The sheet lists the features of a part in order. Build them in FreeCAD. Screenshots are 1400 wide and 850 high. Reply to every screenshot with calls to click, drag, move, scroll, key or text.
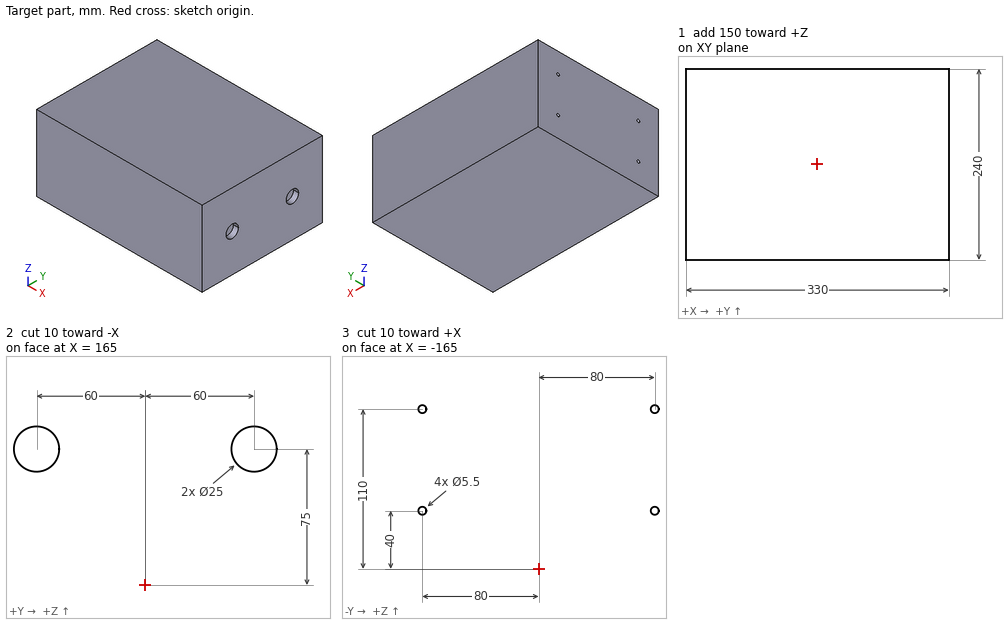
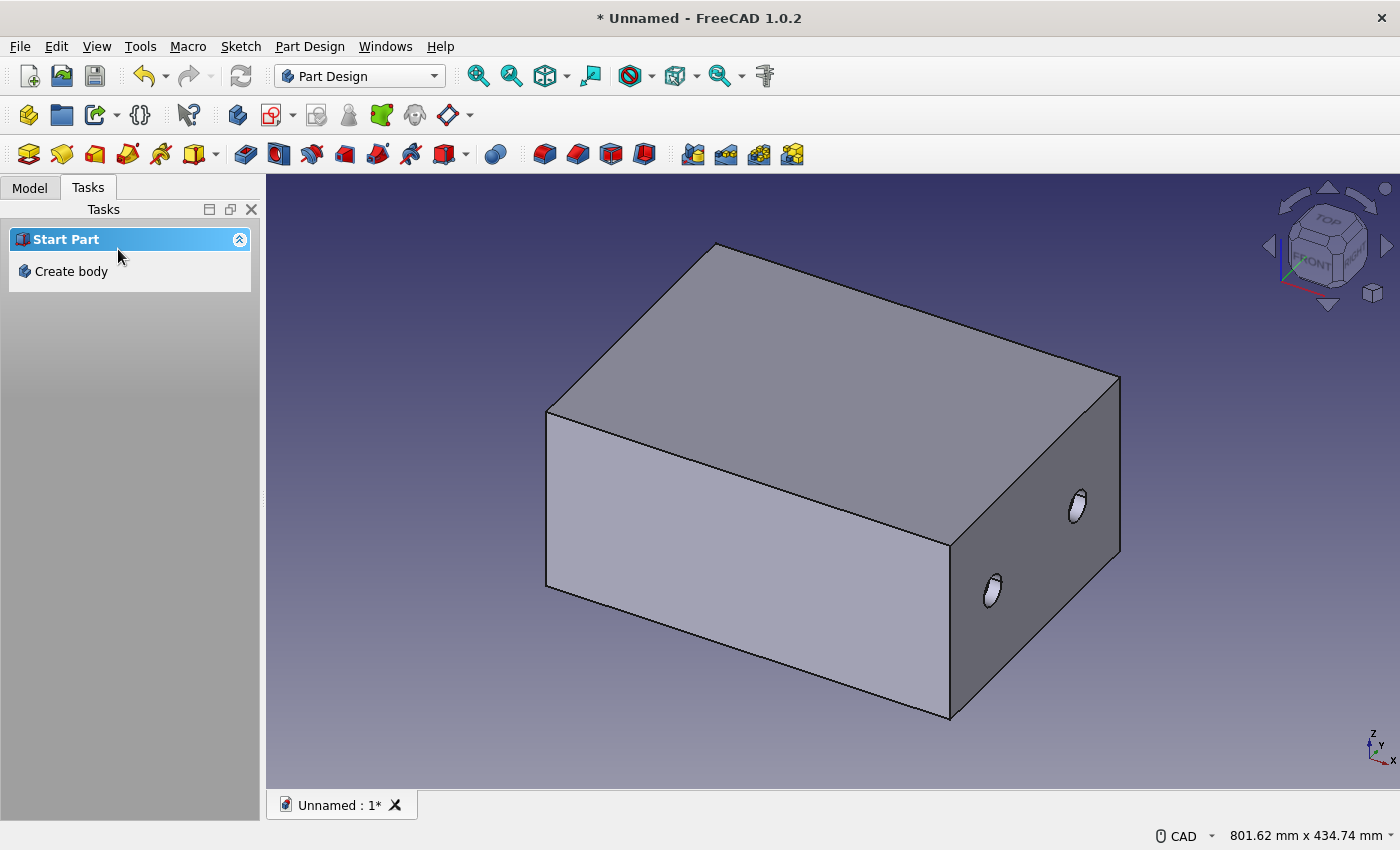
key(6)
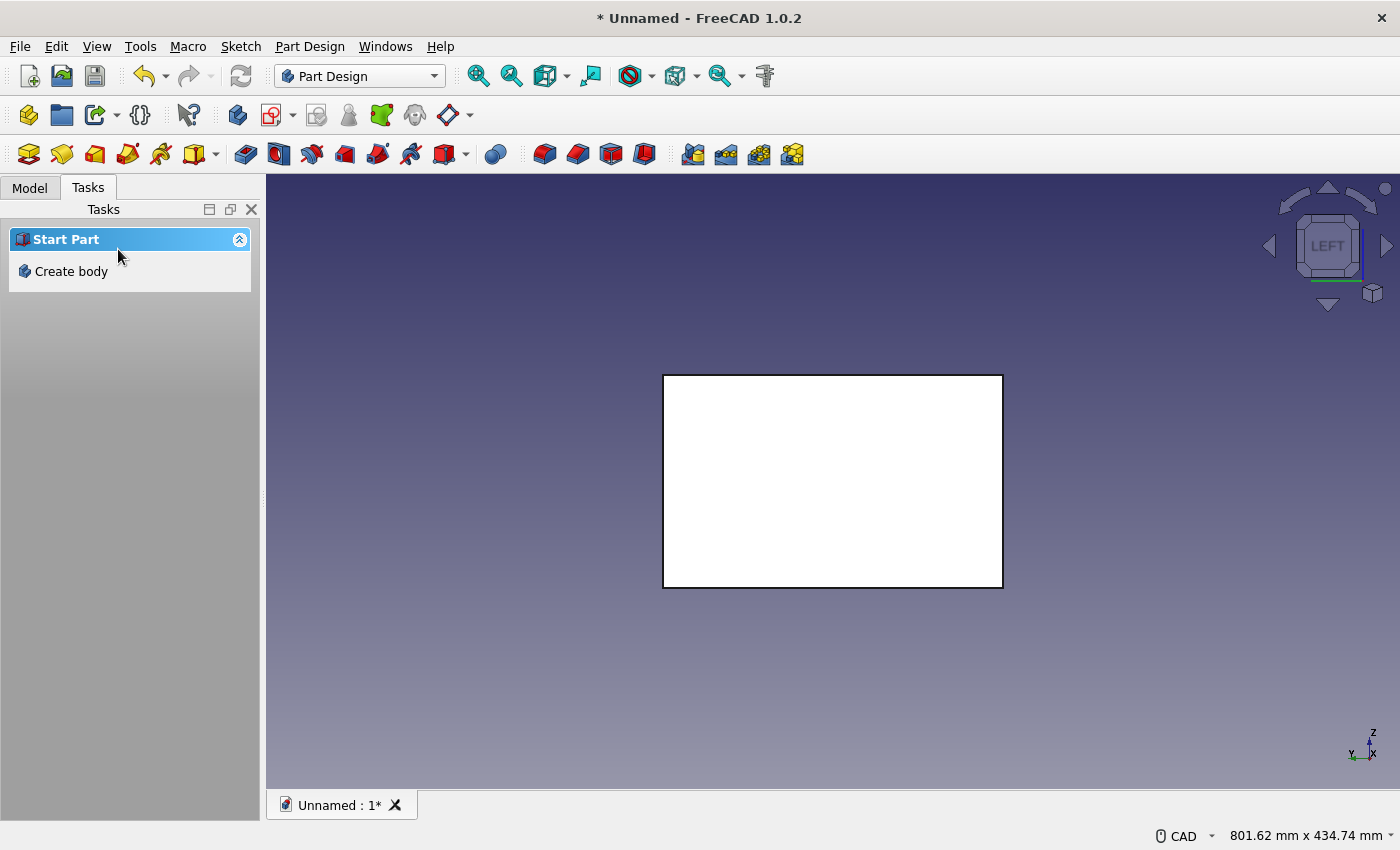
click(479, 76)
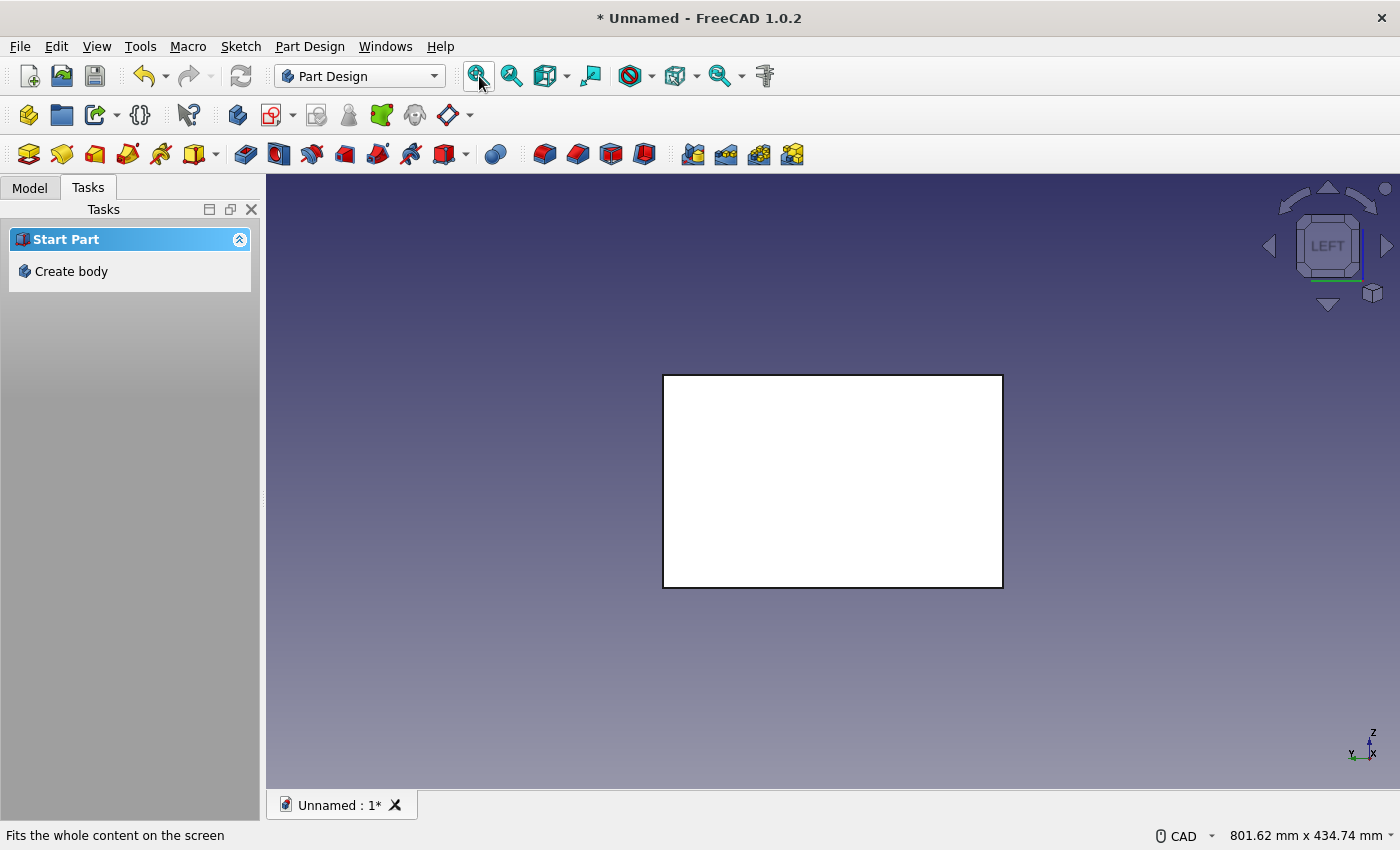
click(784, 480)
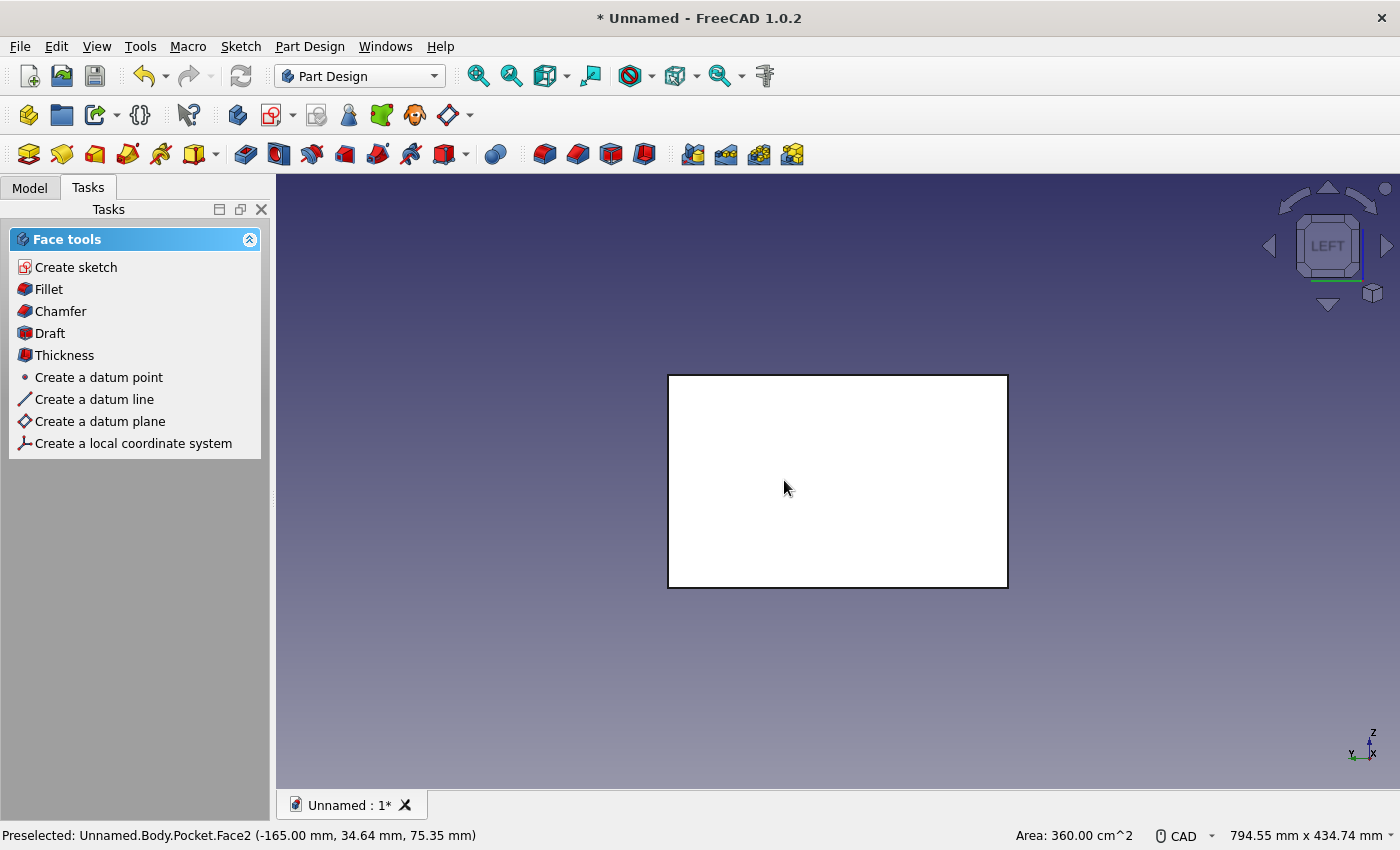
click(270, 116)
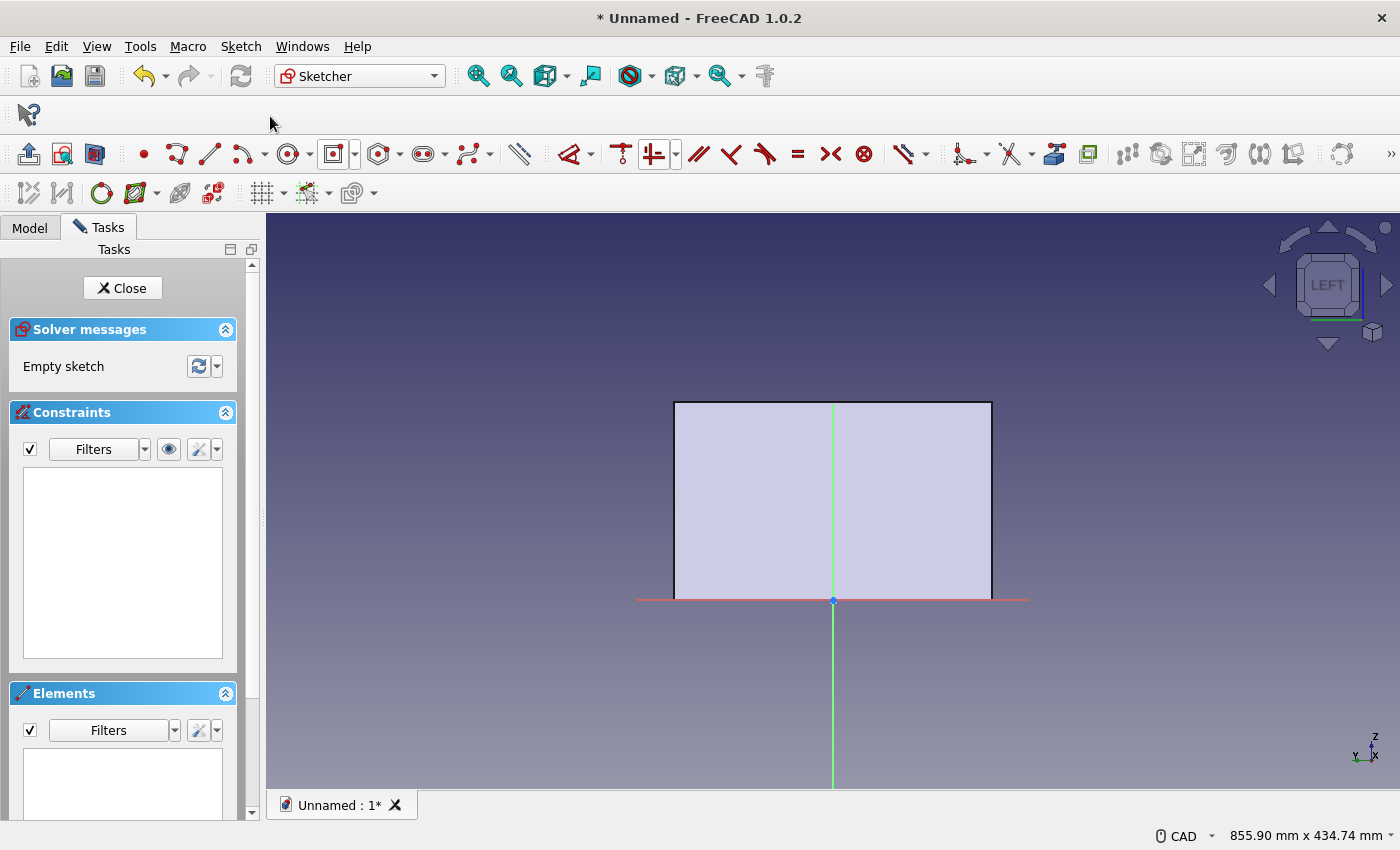
scroll(889, 546, up, 4)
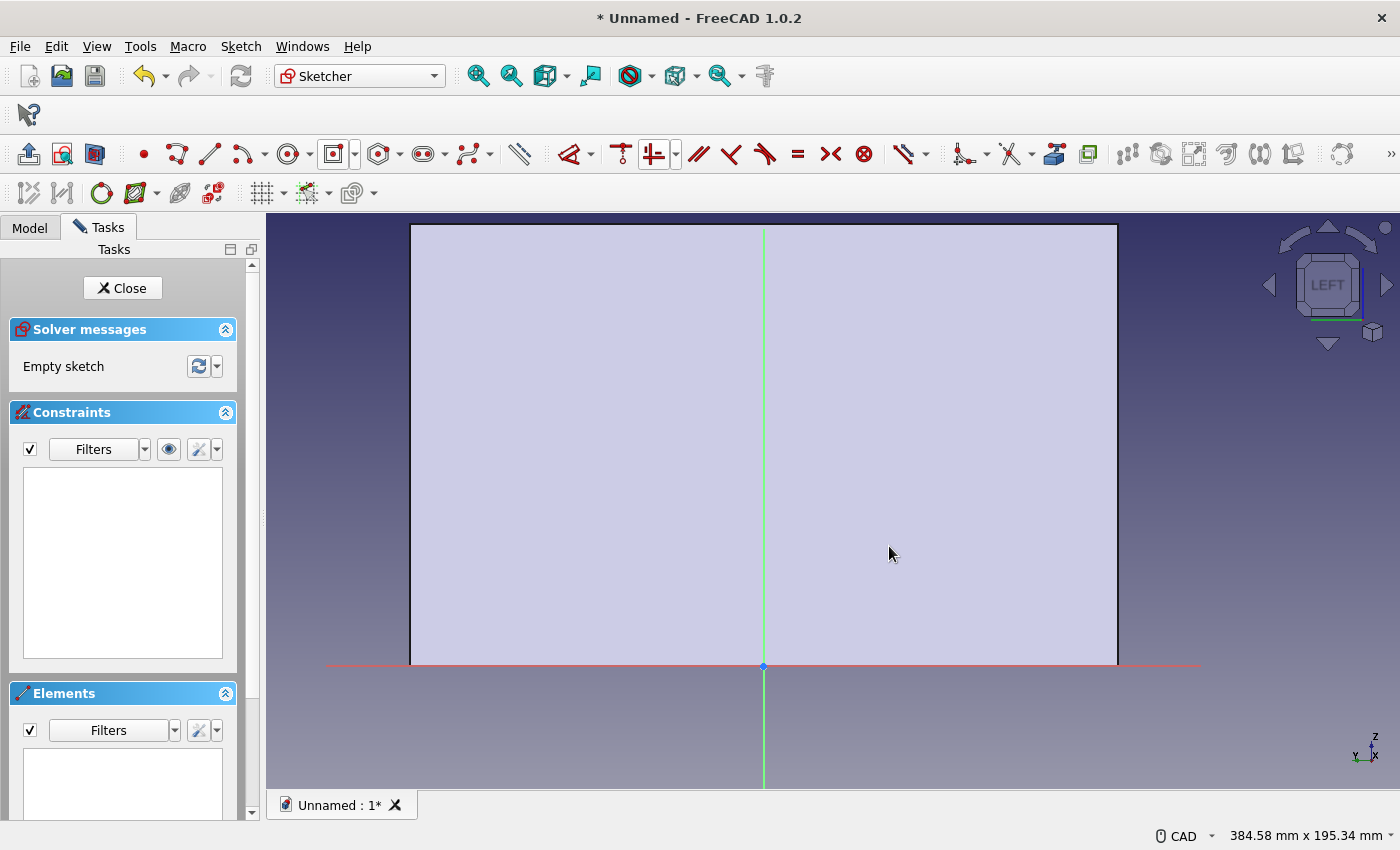
click(288, 154)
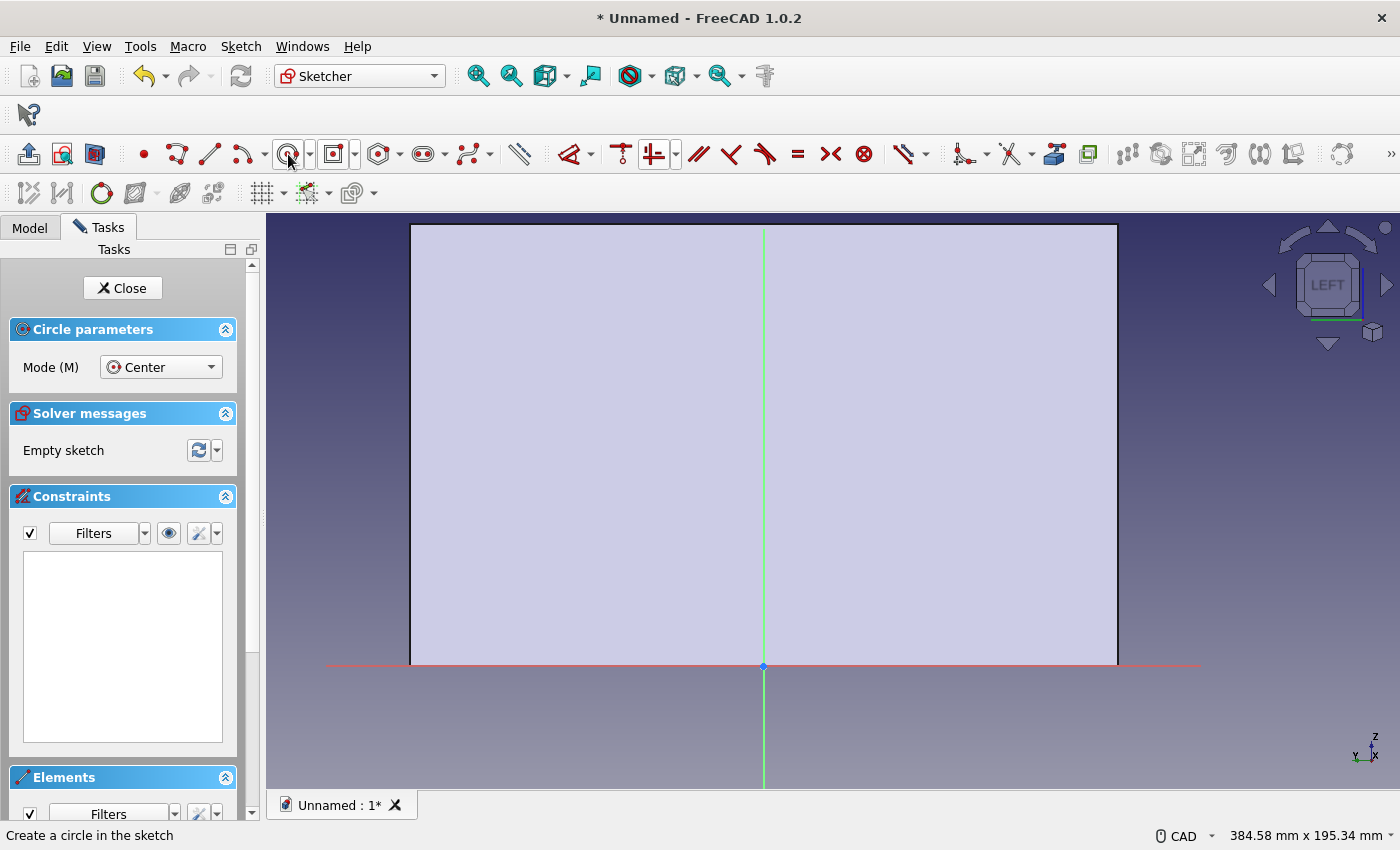
scroll(528, 548, up, 6)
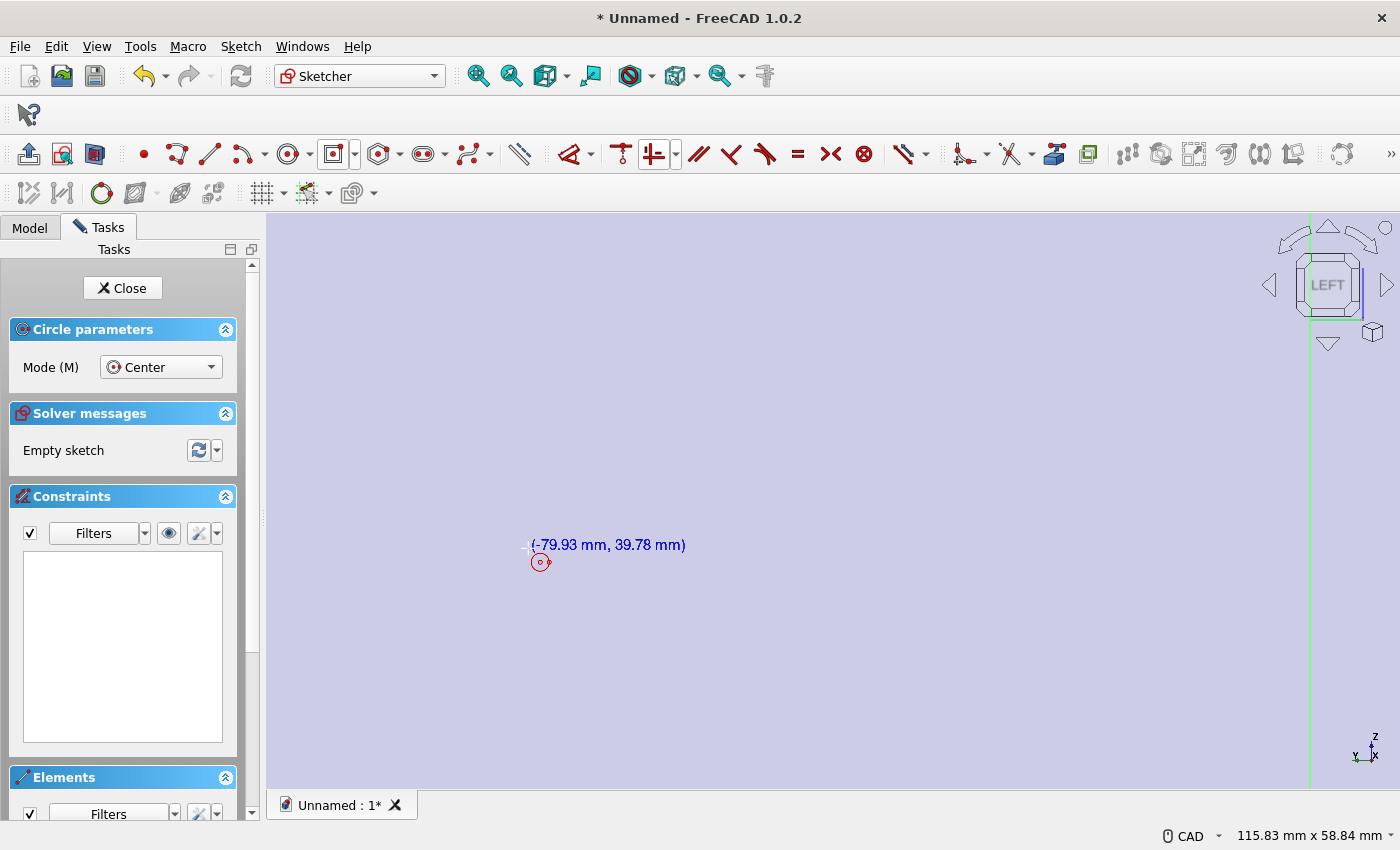
click(527, 548)
move(546, 529)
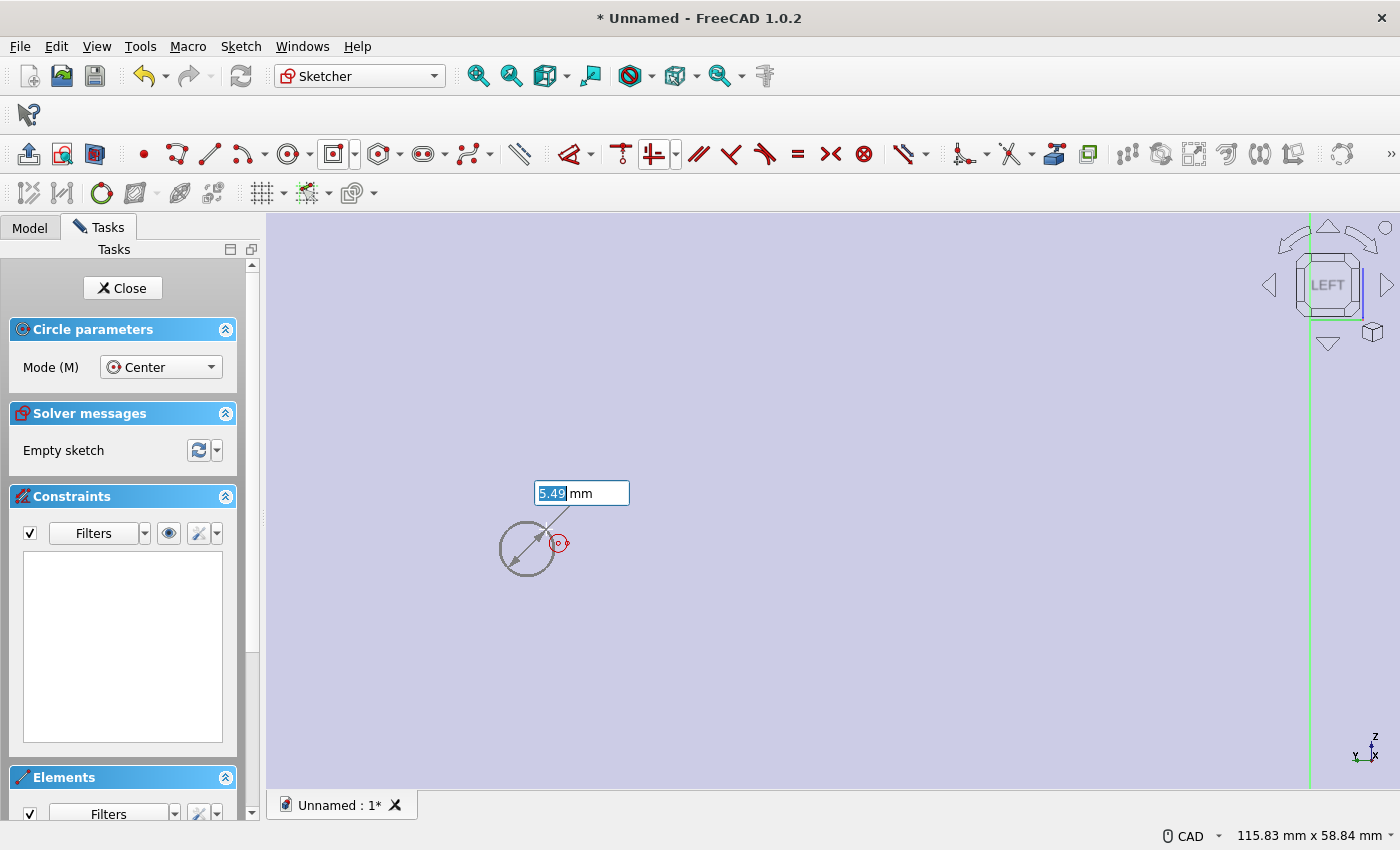
text(5.5)
key(Return)